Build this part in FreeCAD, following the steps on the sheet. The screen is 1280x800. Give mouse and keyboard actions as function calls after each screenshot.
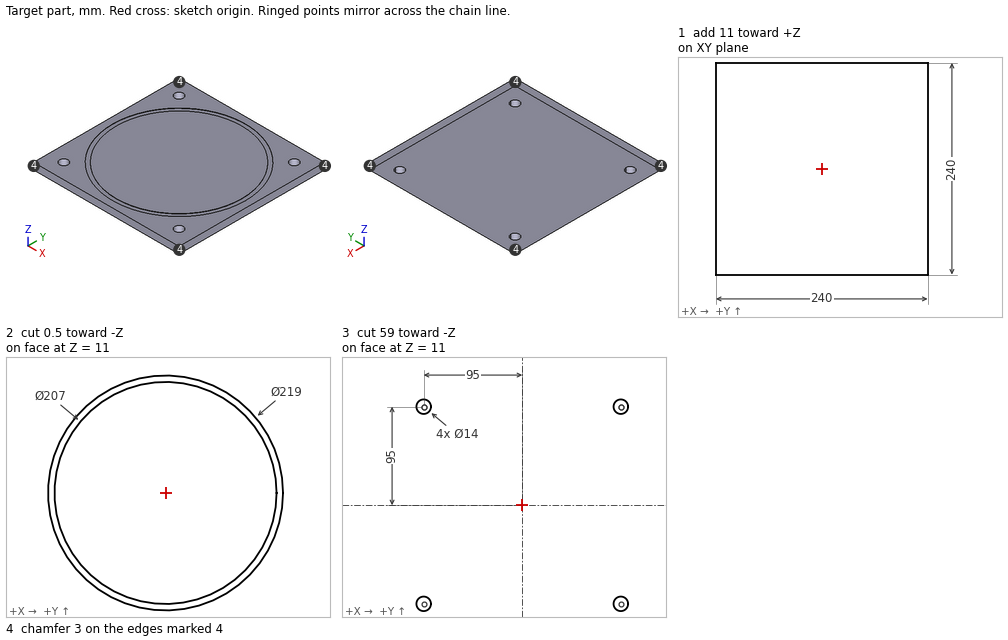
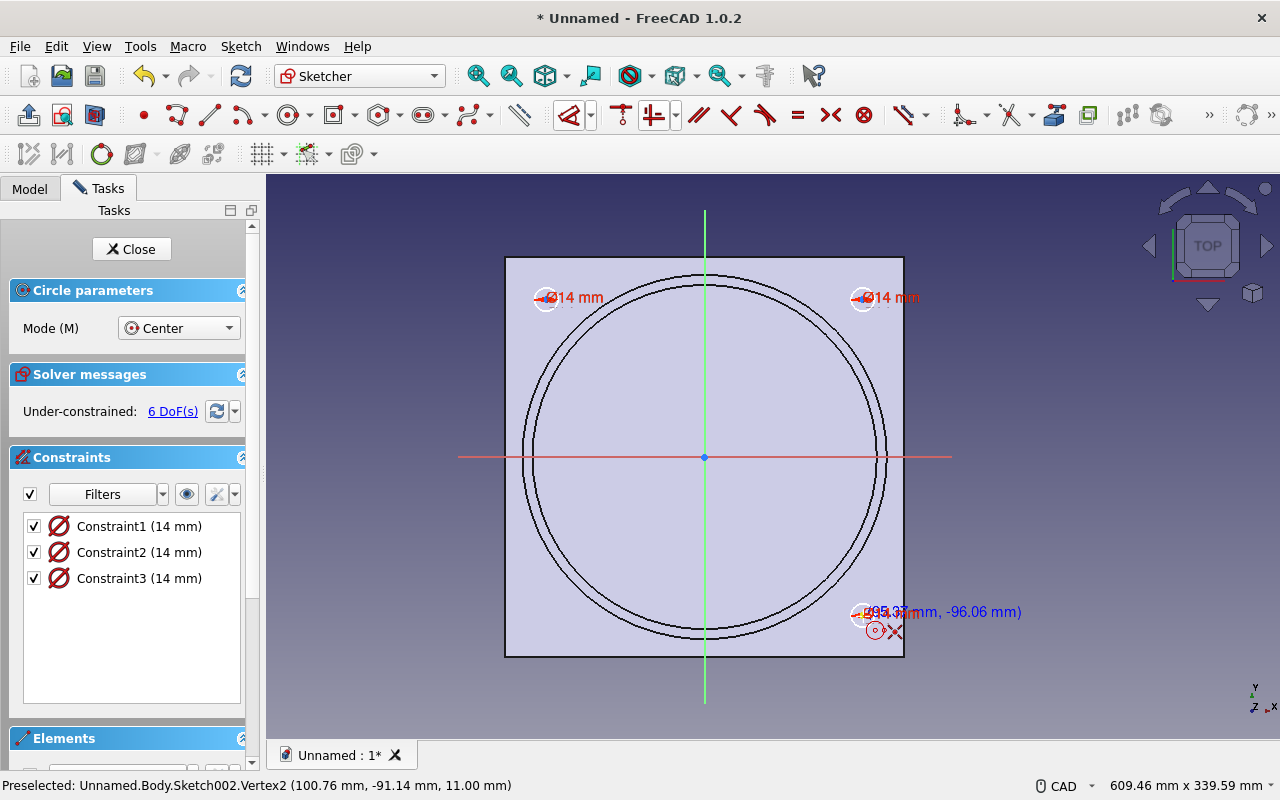
scroll(547, 615, up, 4)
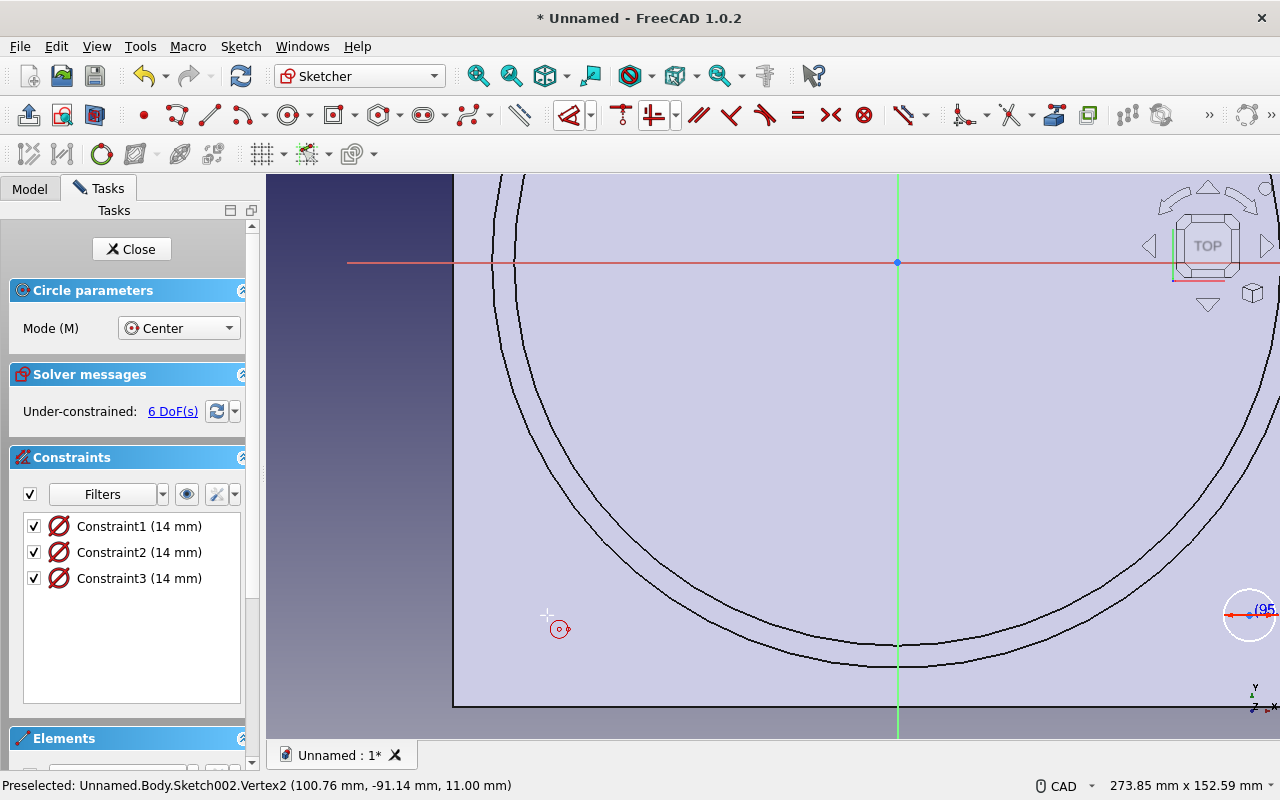
click(546, 614)
move(564, 596)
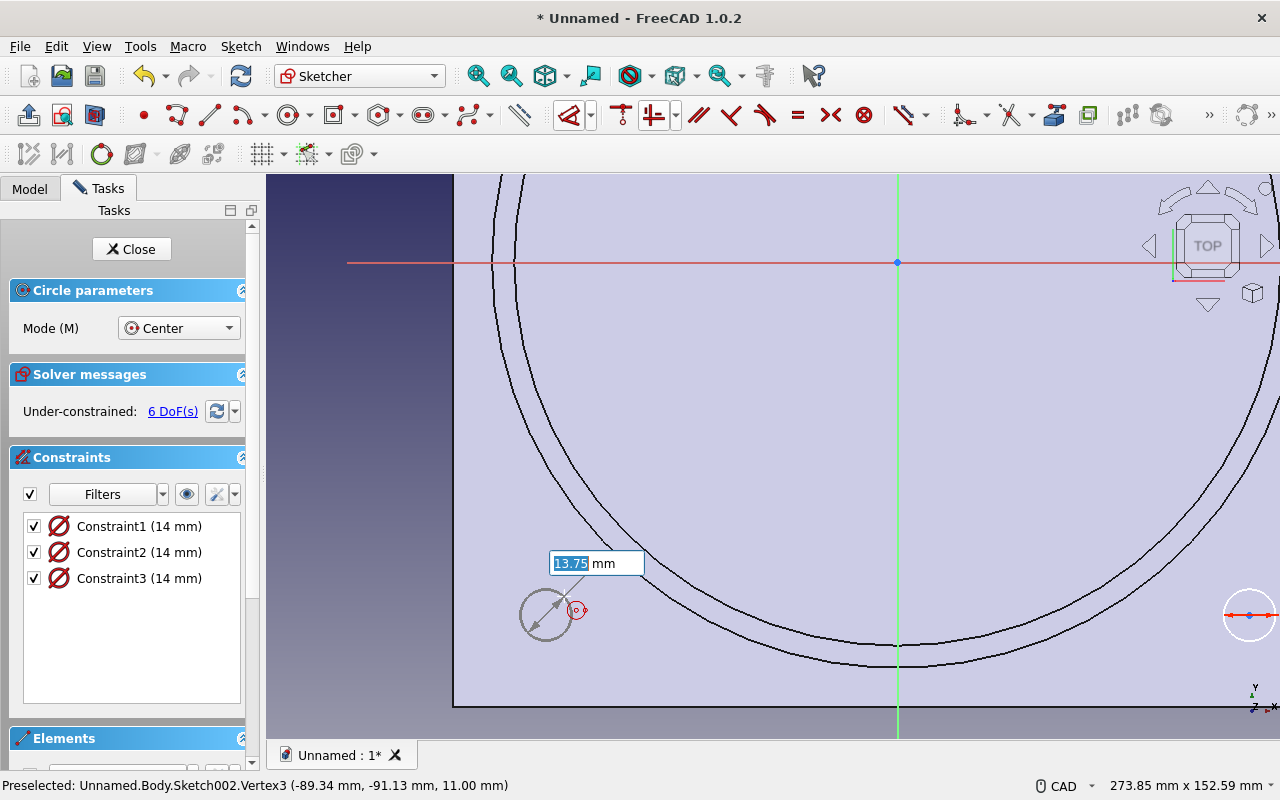
text(14)
key(Return)
key(Escape)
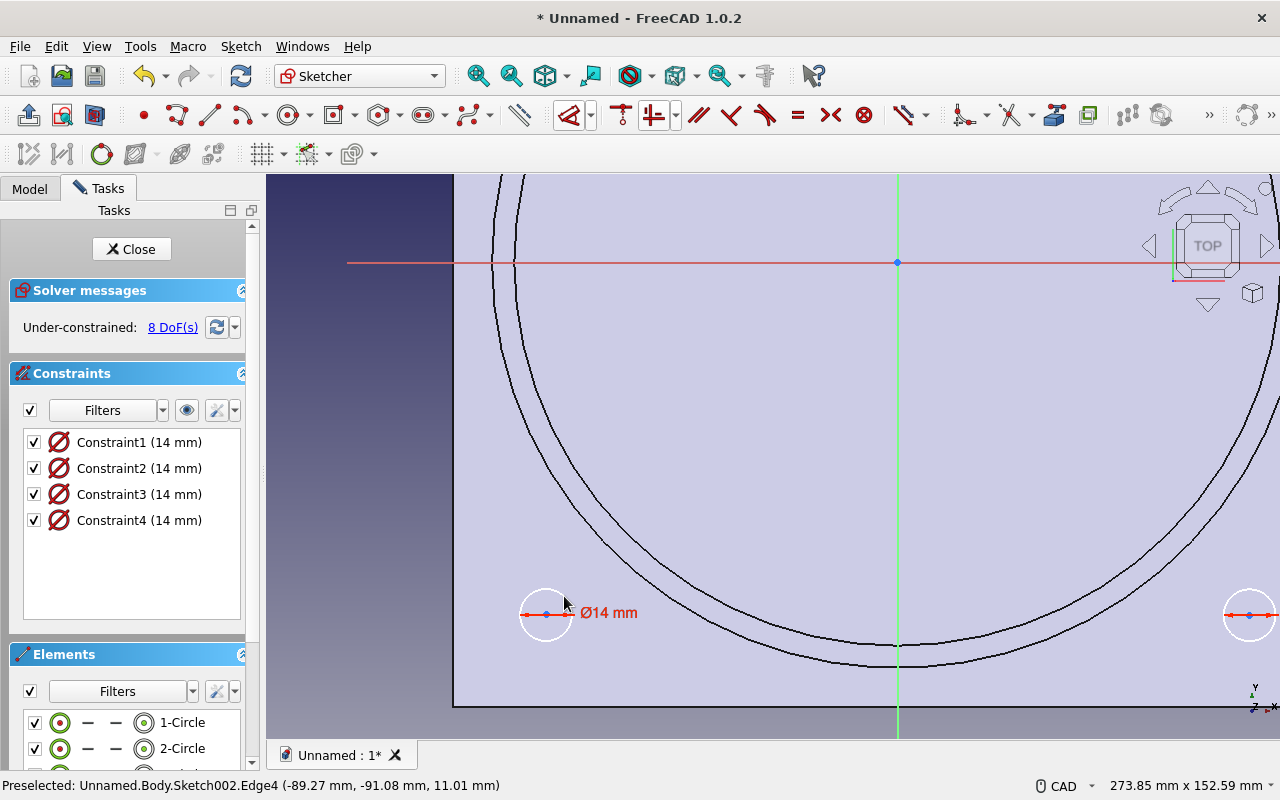
scroll(547, 615, down, 4)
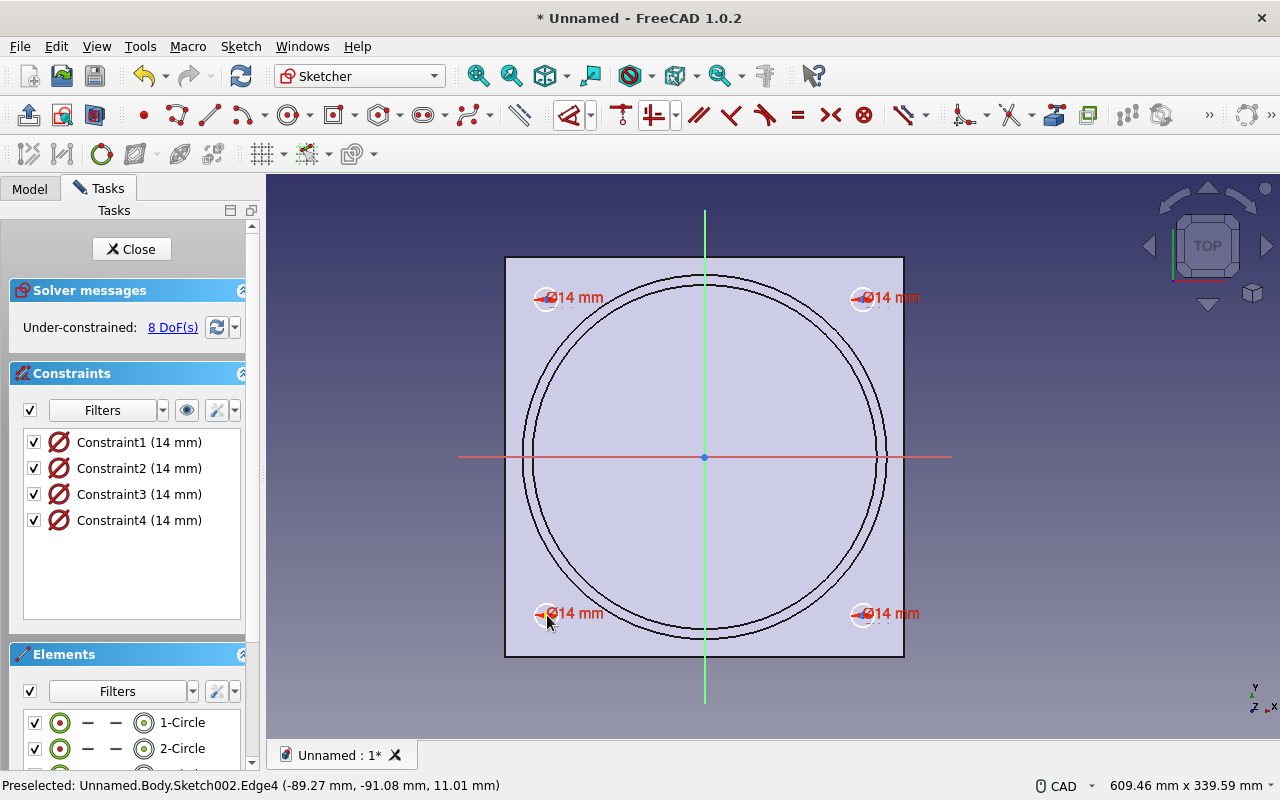
click(546, 300)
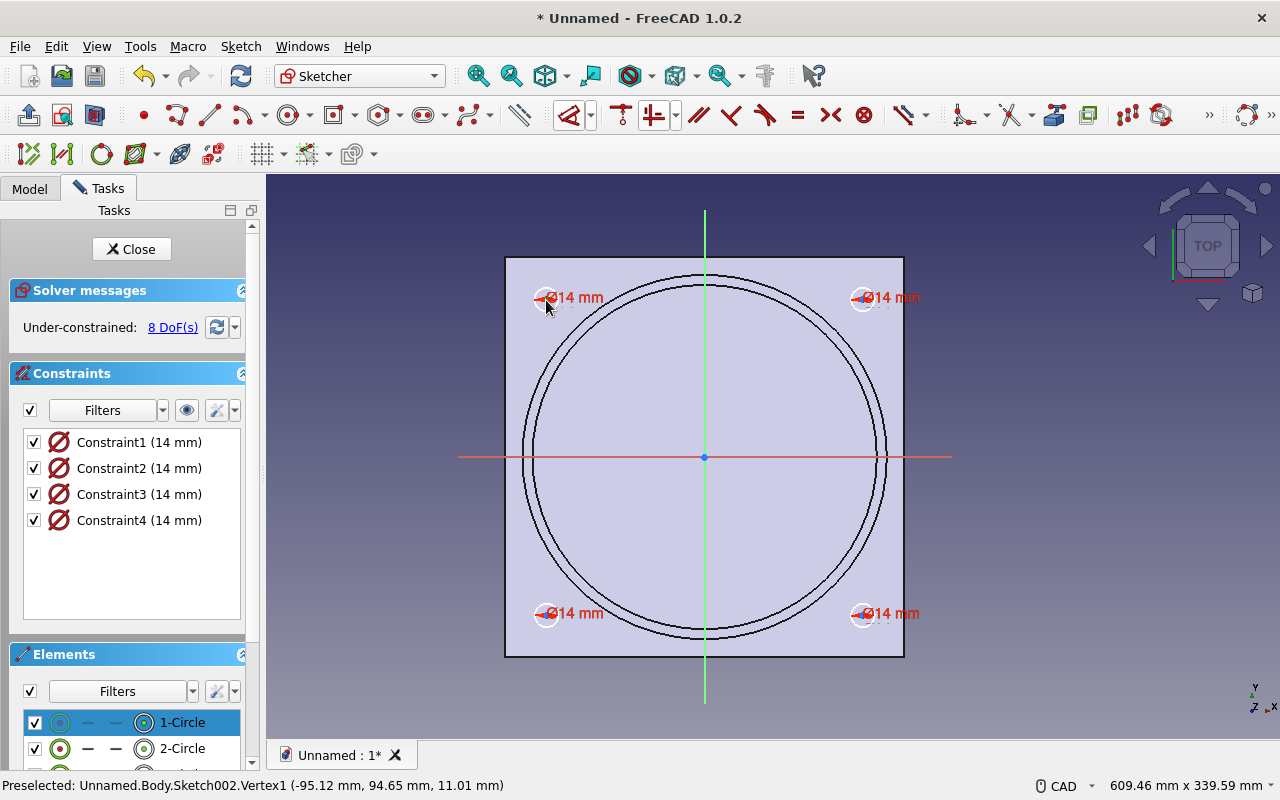
click(863, 300)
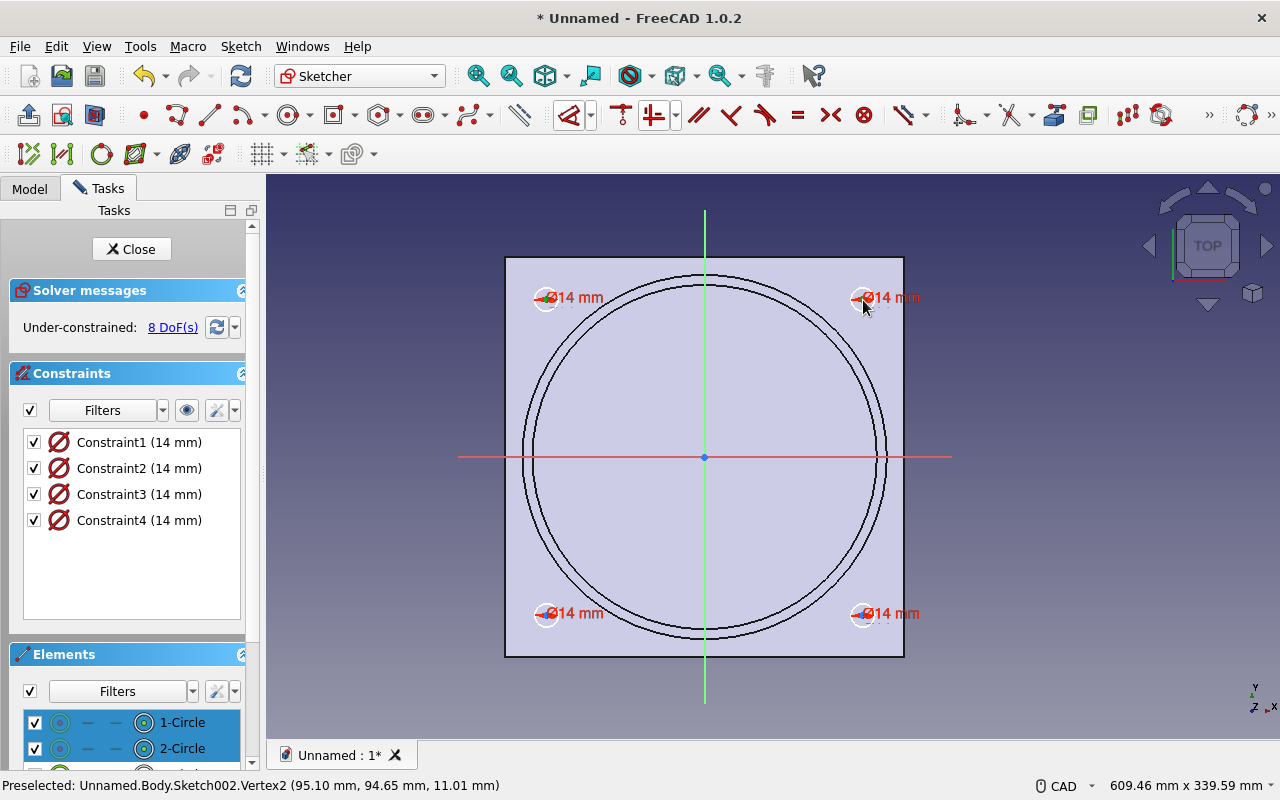
click(705, 675)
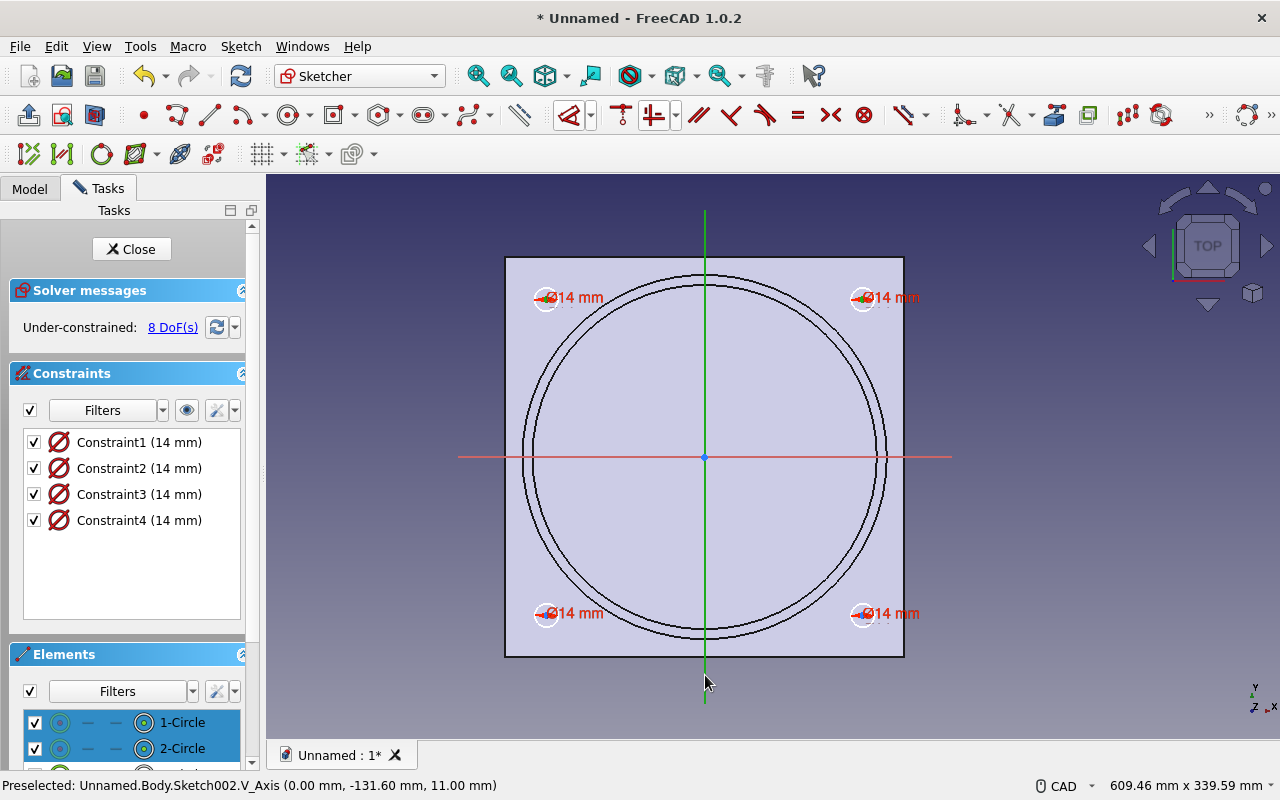
click(831, 116)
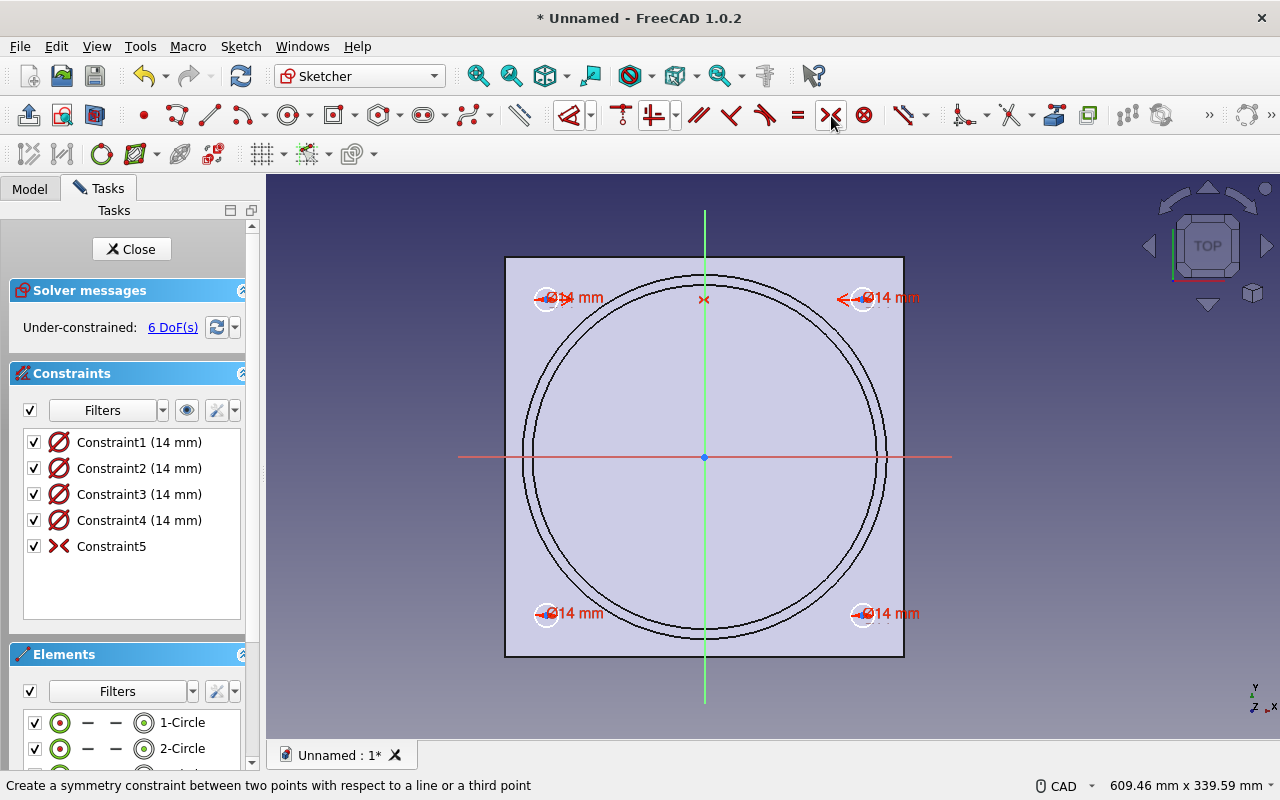
click(863, 300)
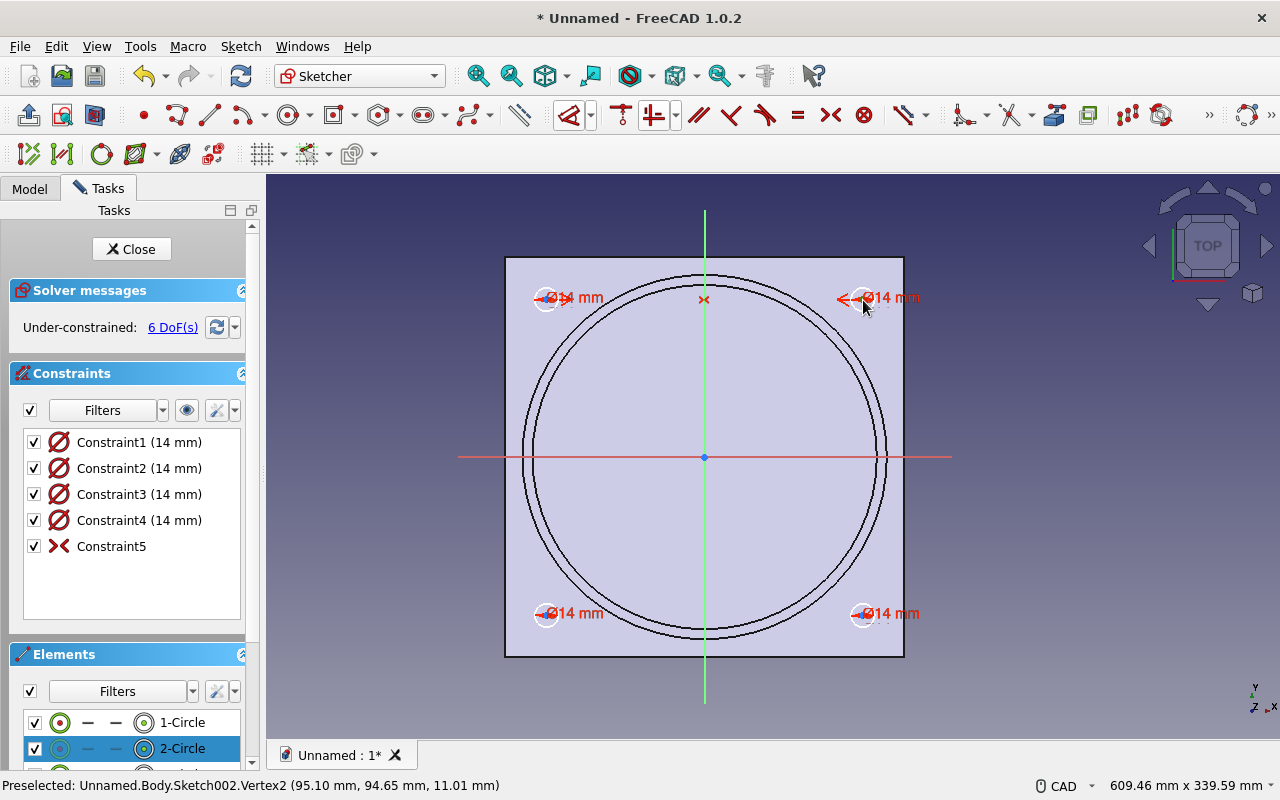
click(863, 616)